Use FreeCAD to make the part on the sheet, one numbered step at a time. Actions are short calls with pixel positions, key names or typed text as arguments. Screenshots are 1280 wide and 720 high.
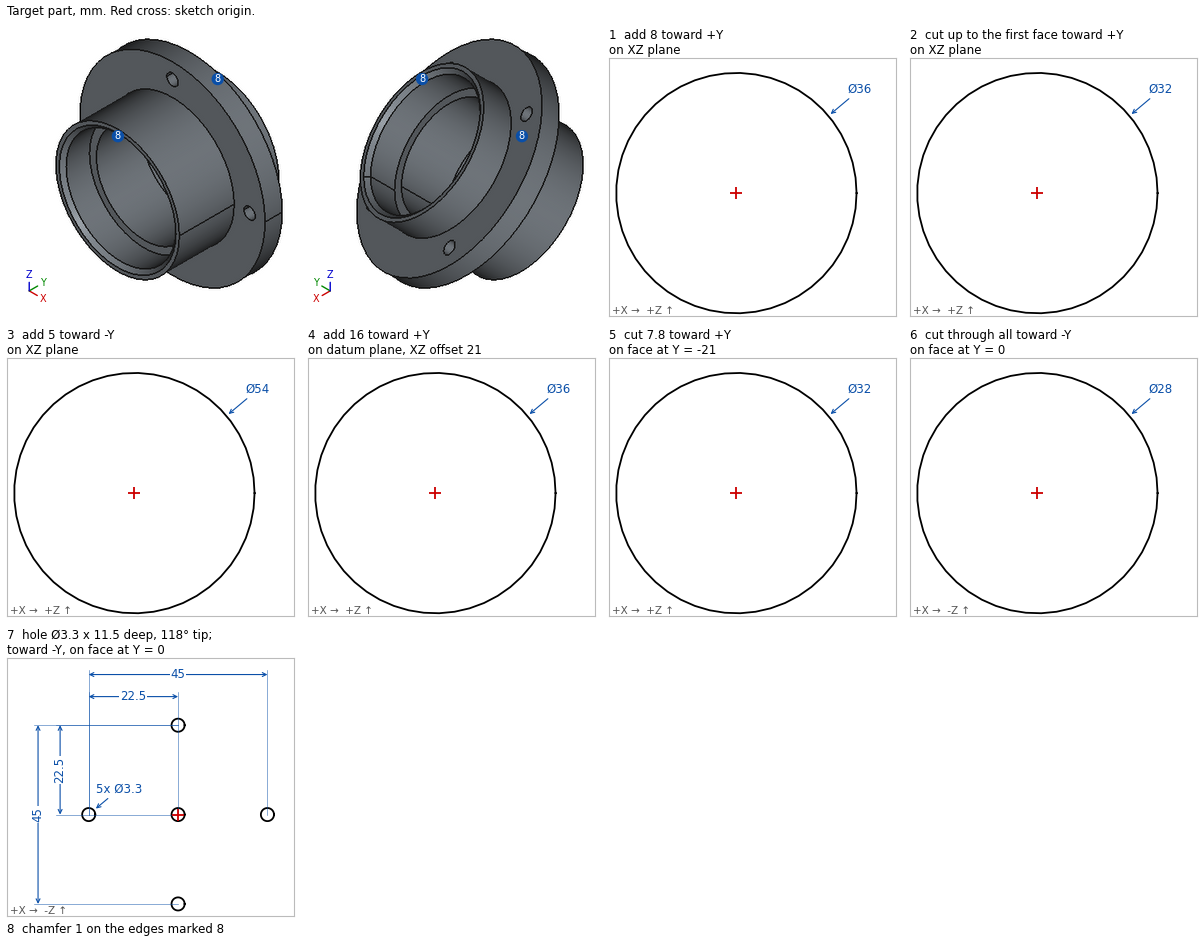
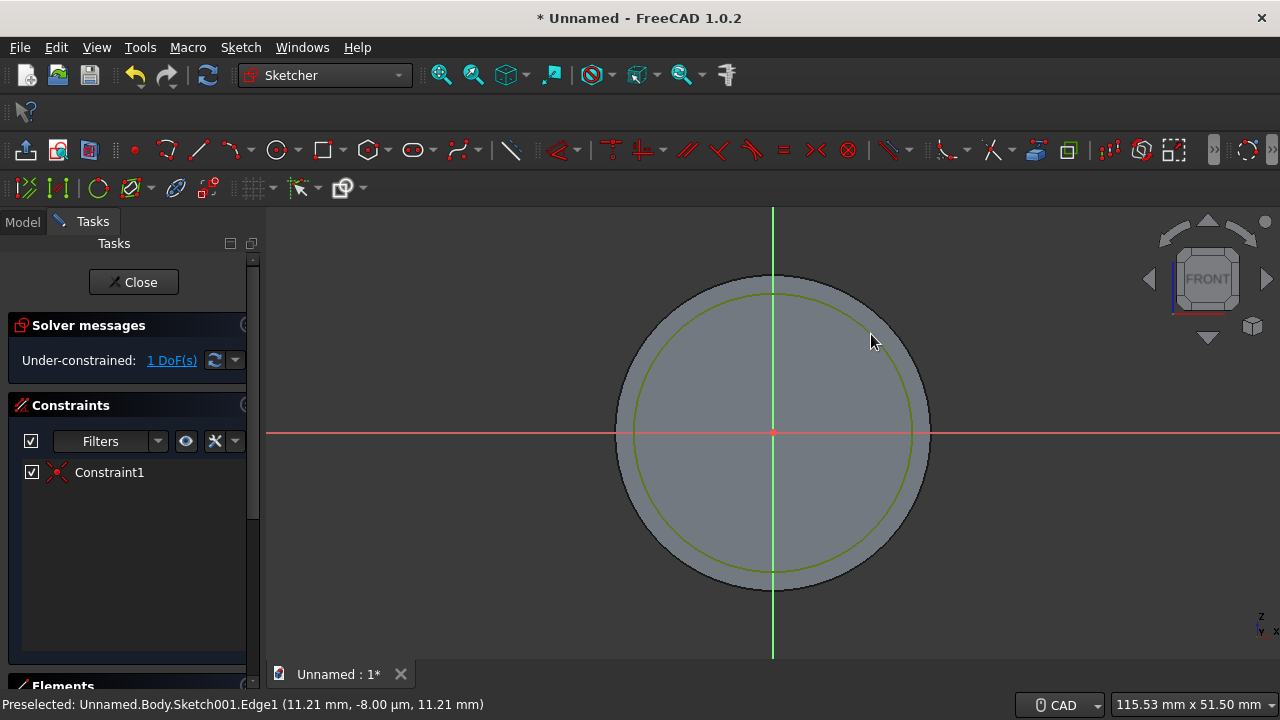
click(580, 150)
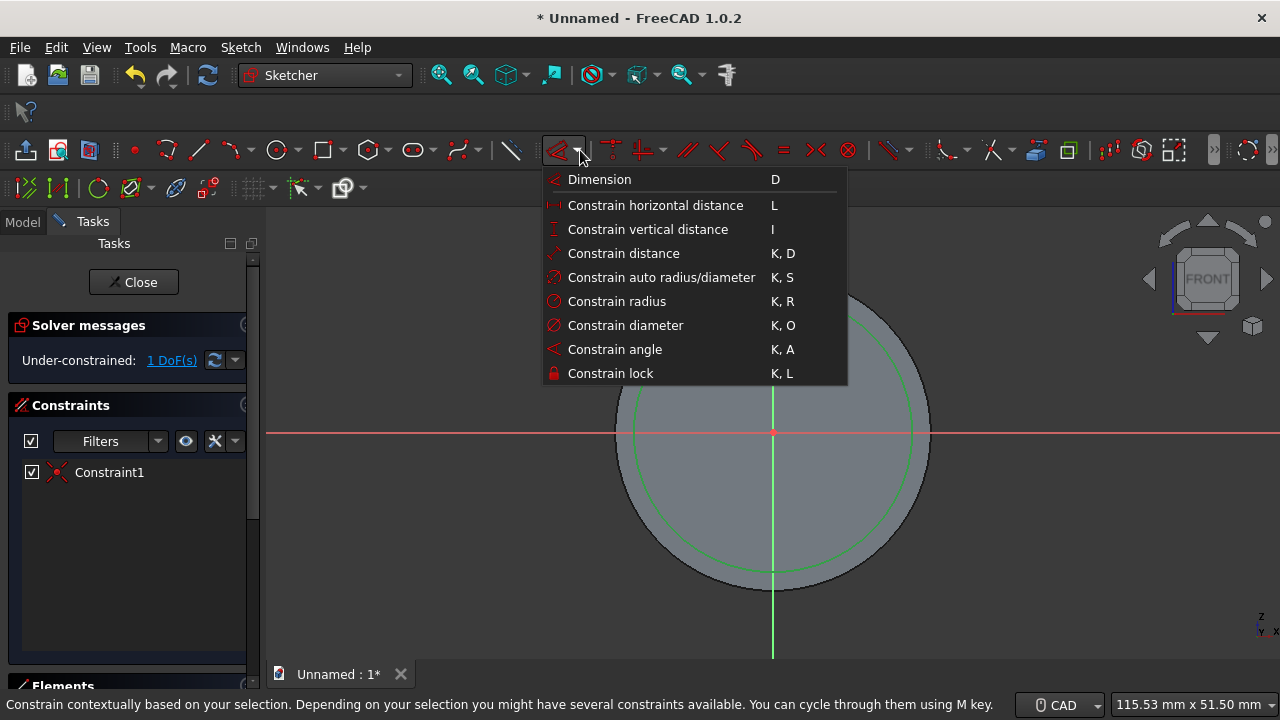
click(695, 325)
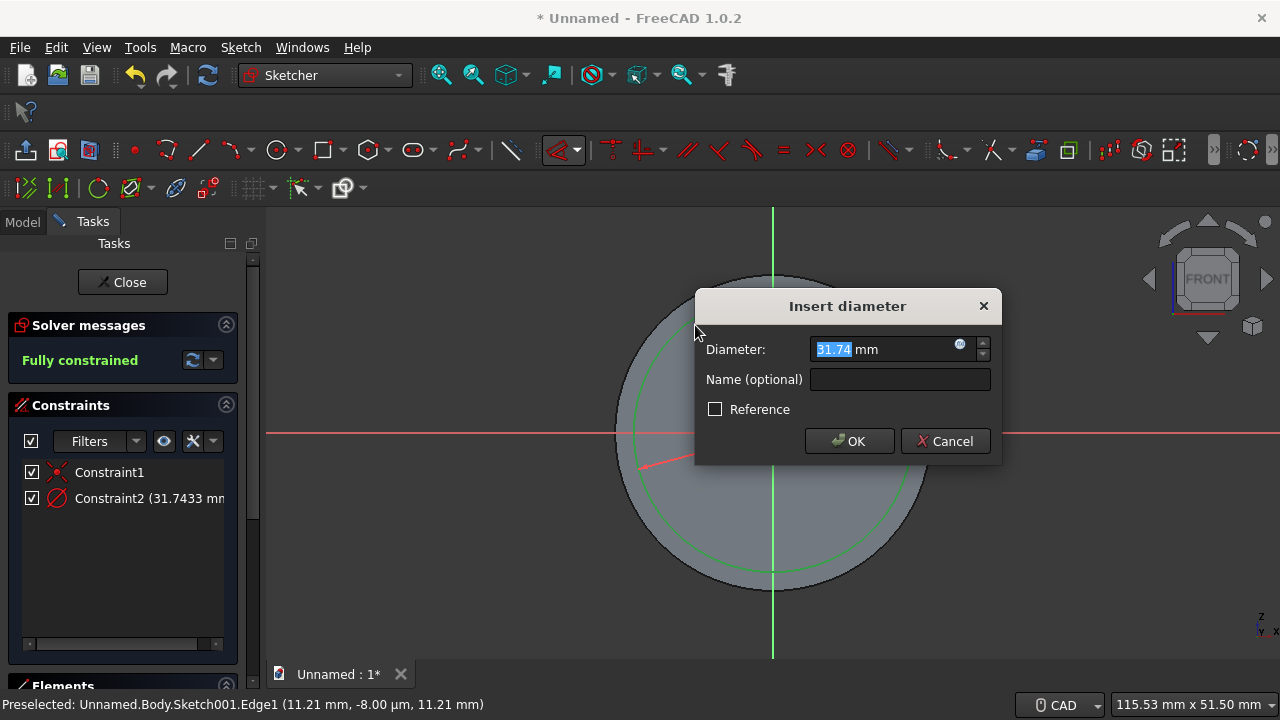
text(32)
key(Return)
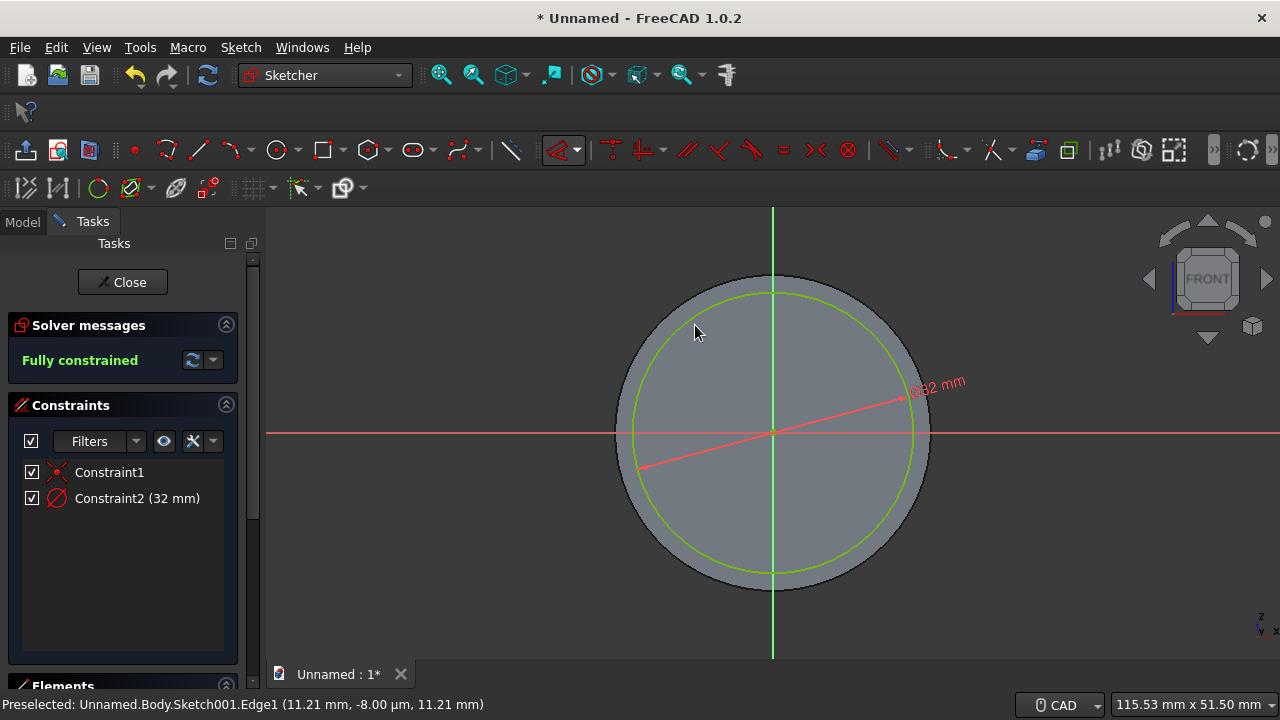
click(123, 282)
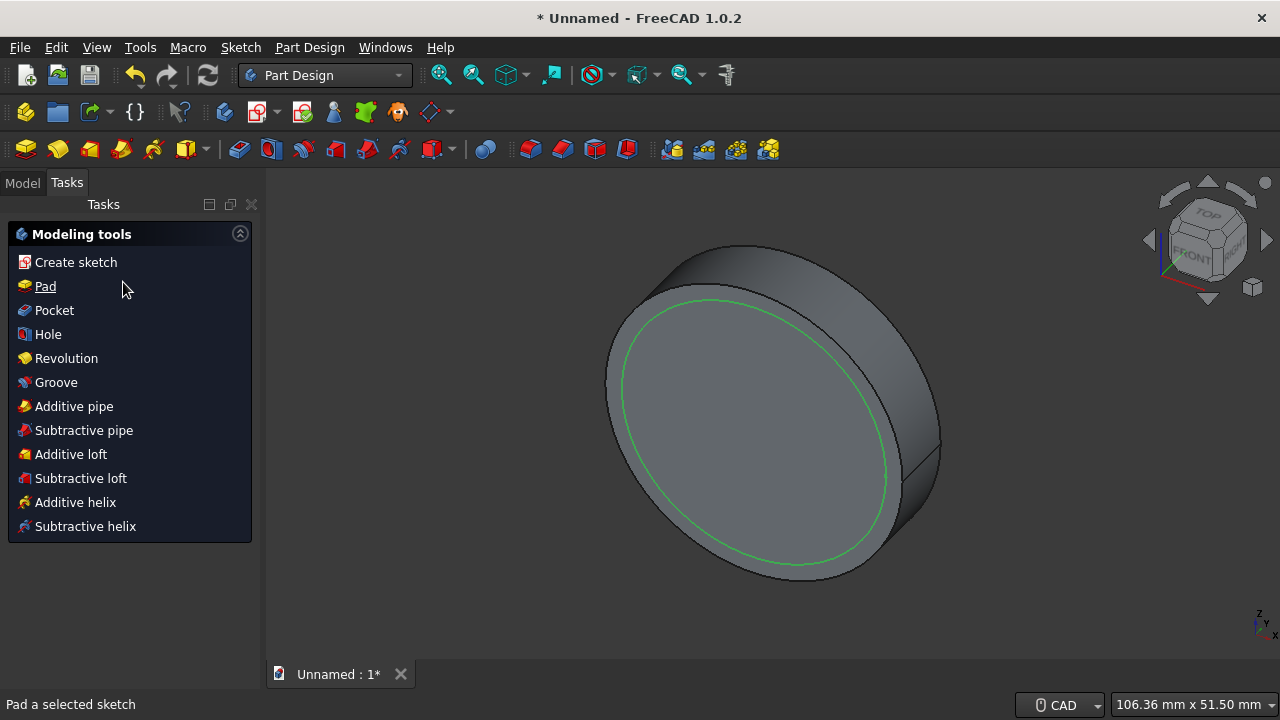
click(240, 150)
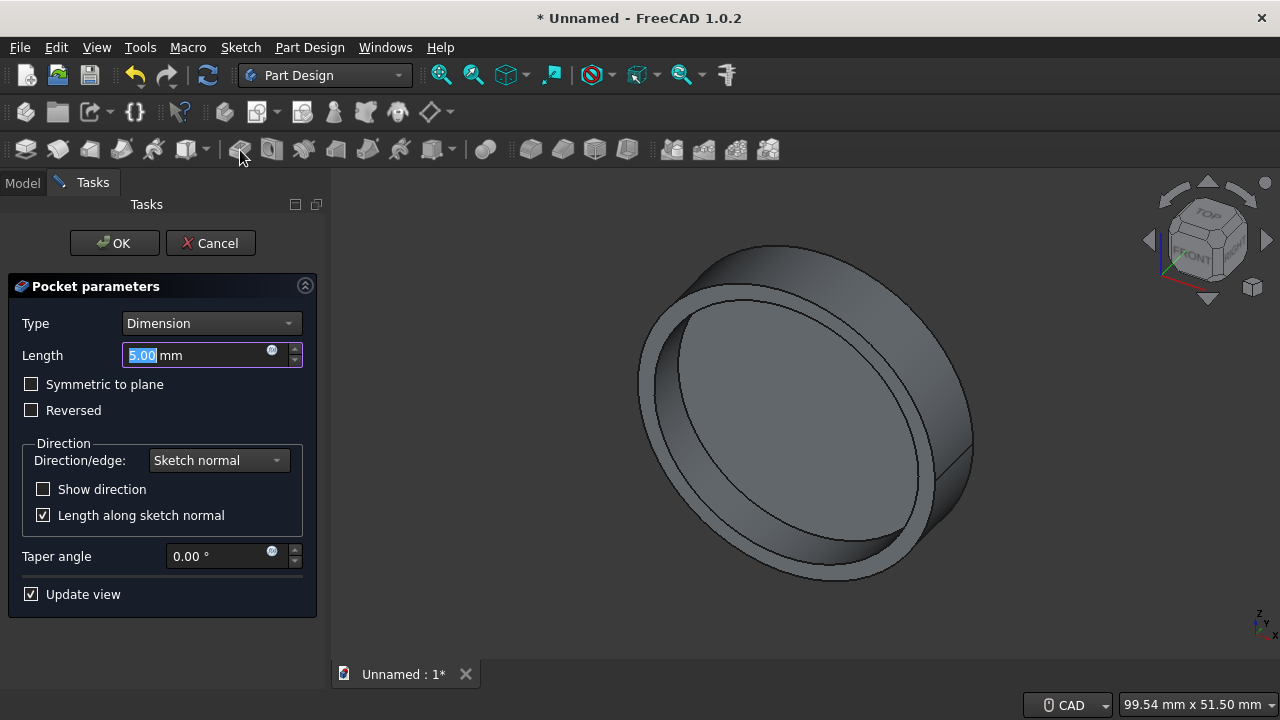
click(212, 324)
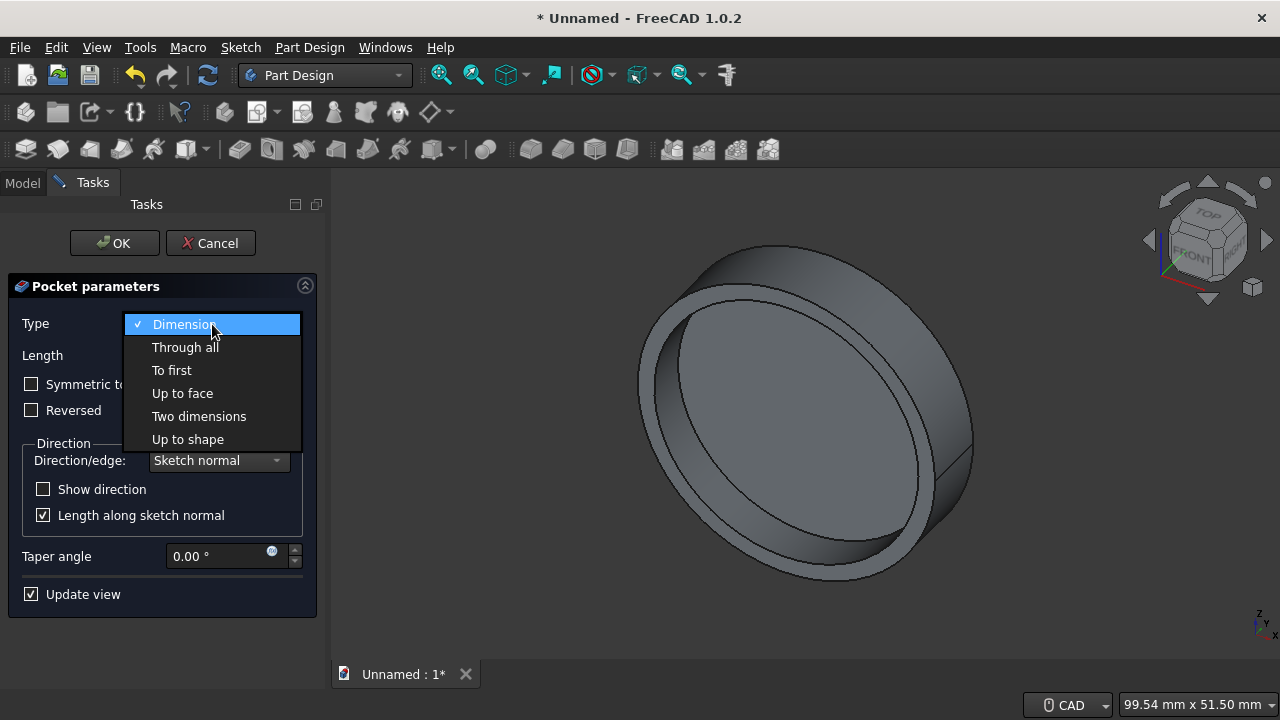
click(212, 370)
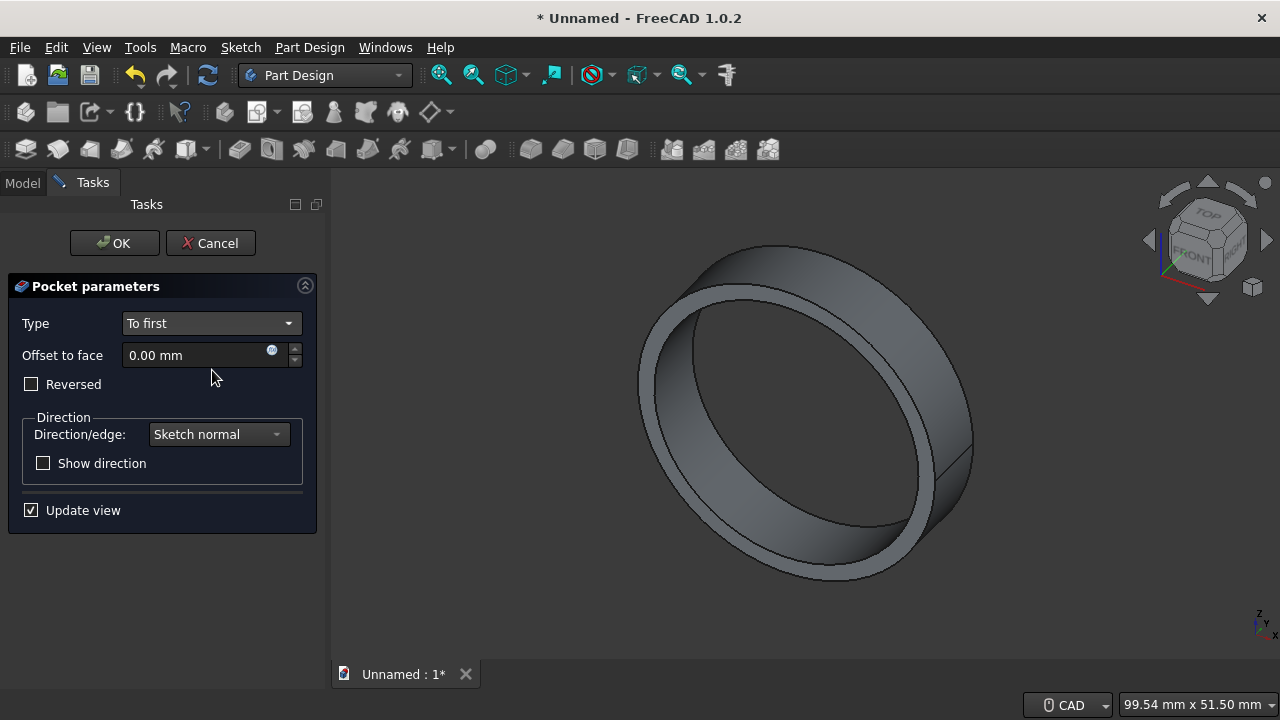
click(115, 243)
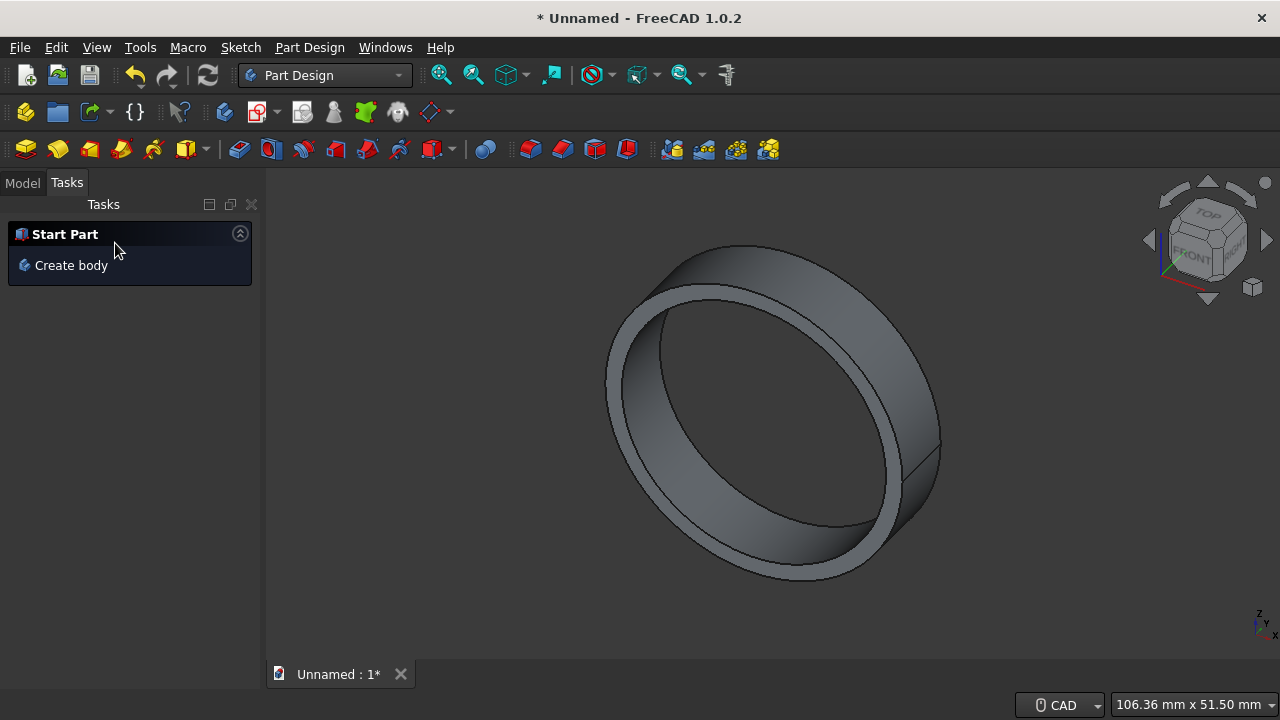
click(258, 112)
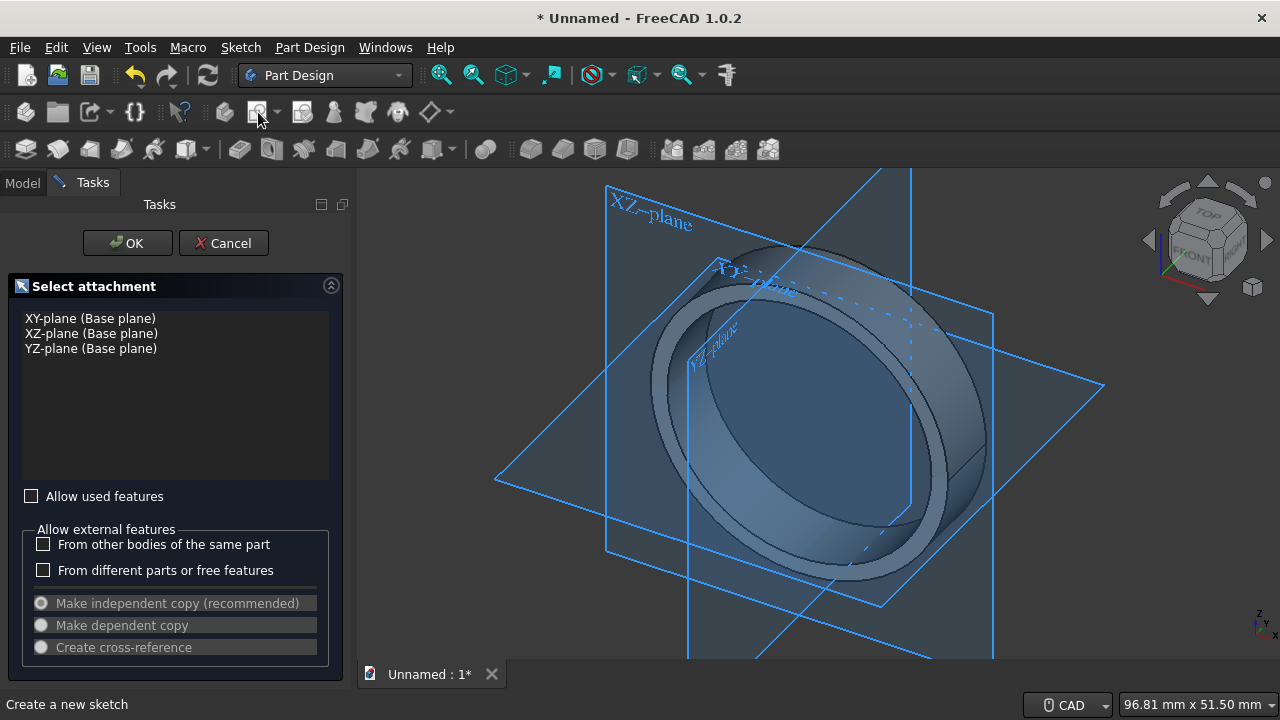
click(82, 334)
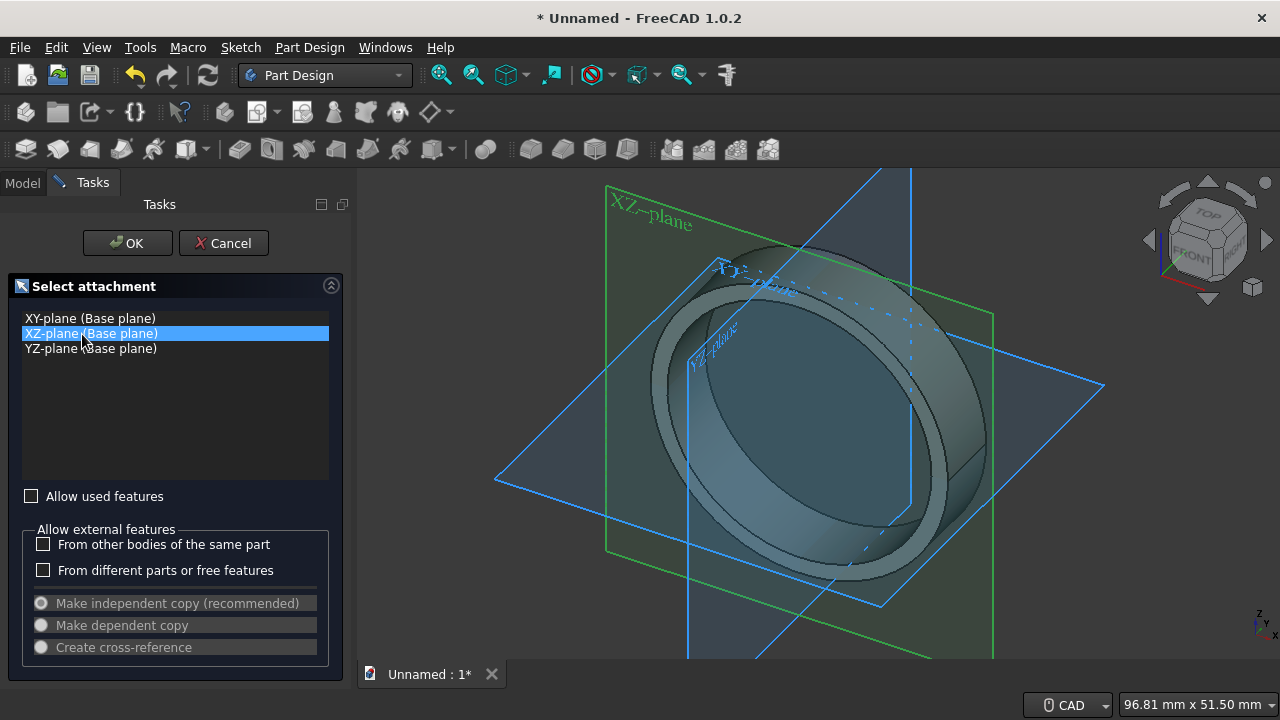
click(128, 243)